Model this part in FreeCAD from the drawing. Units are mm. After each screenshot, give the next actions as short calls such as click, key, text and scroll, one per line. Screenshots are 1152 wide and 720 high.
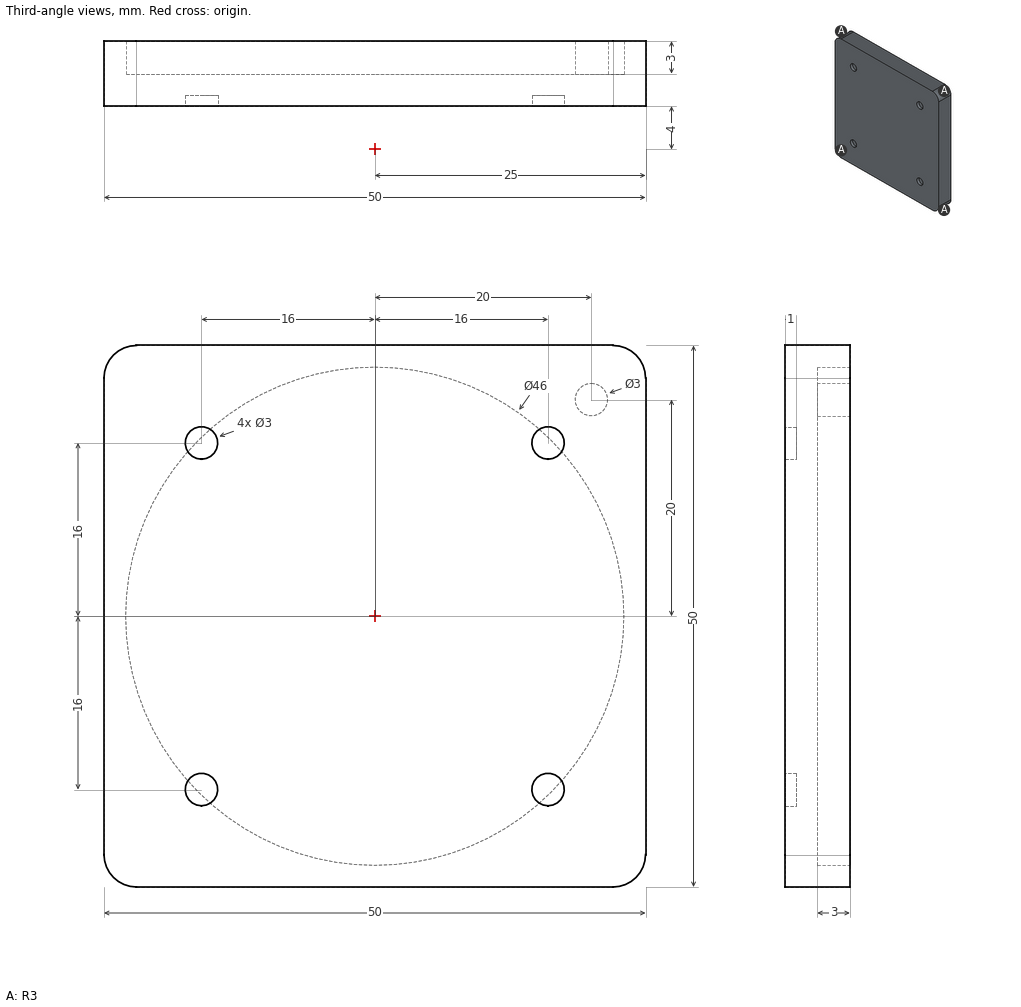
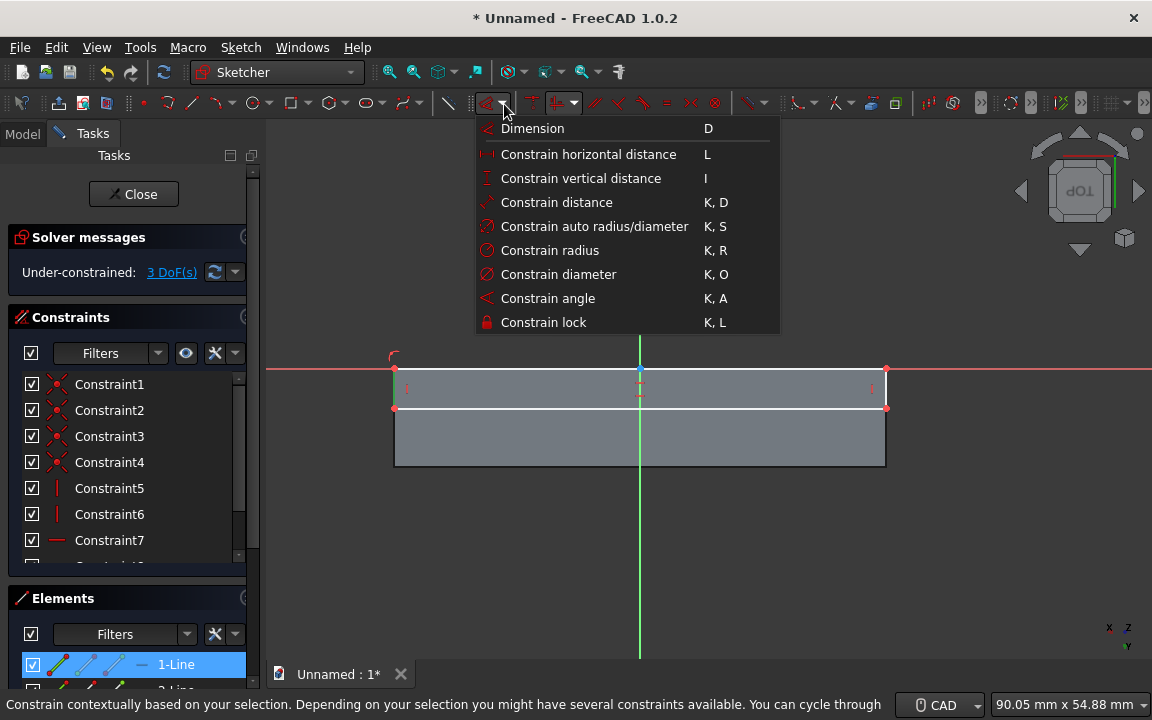
click(628, 178)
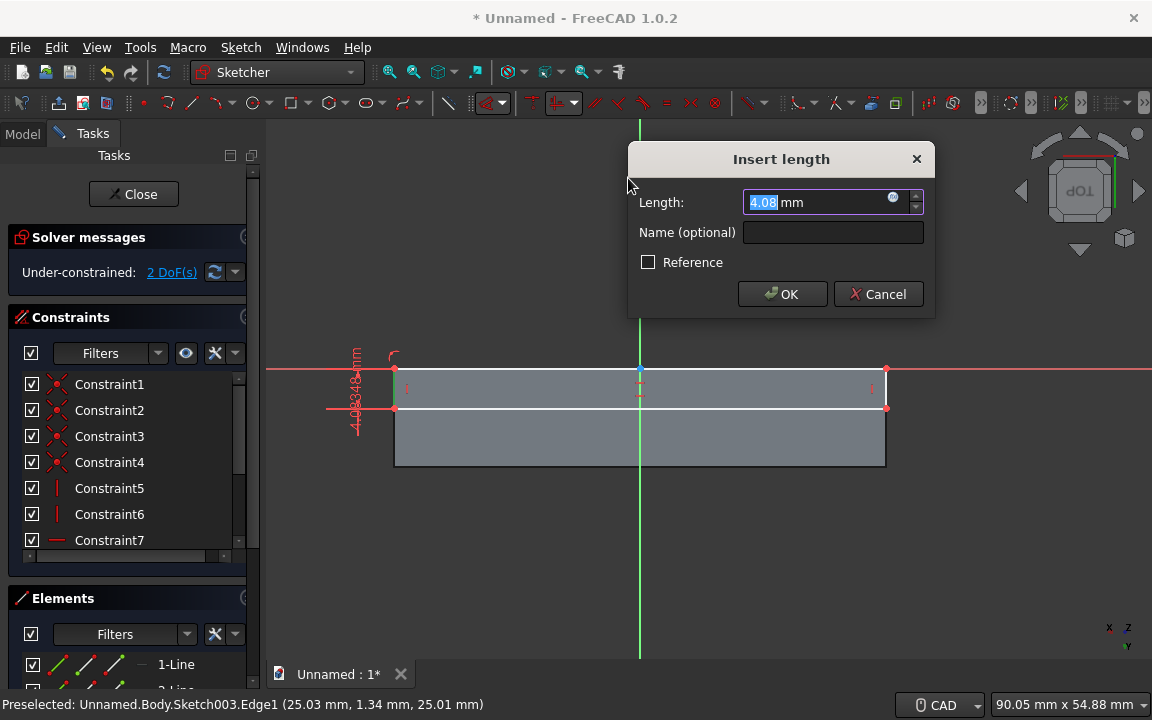
text(4)
key(Return)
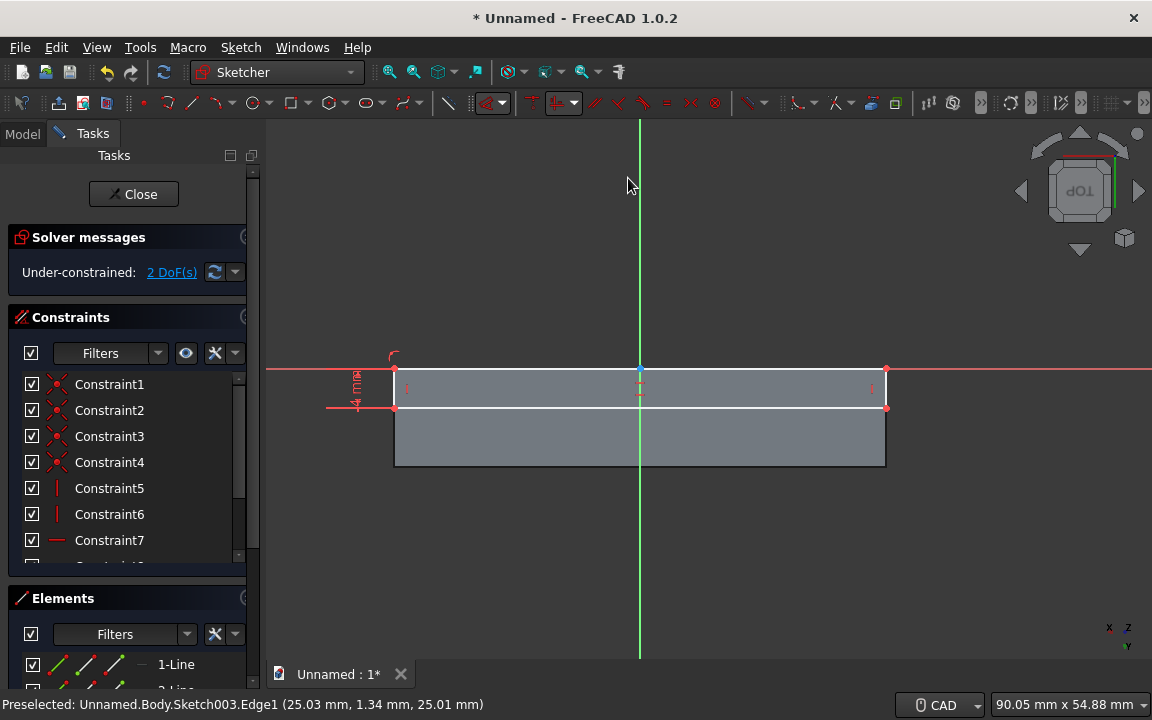
click(542, 408)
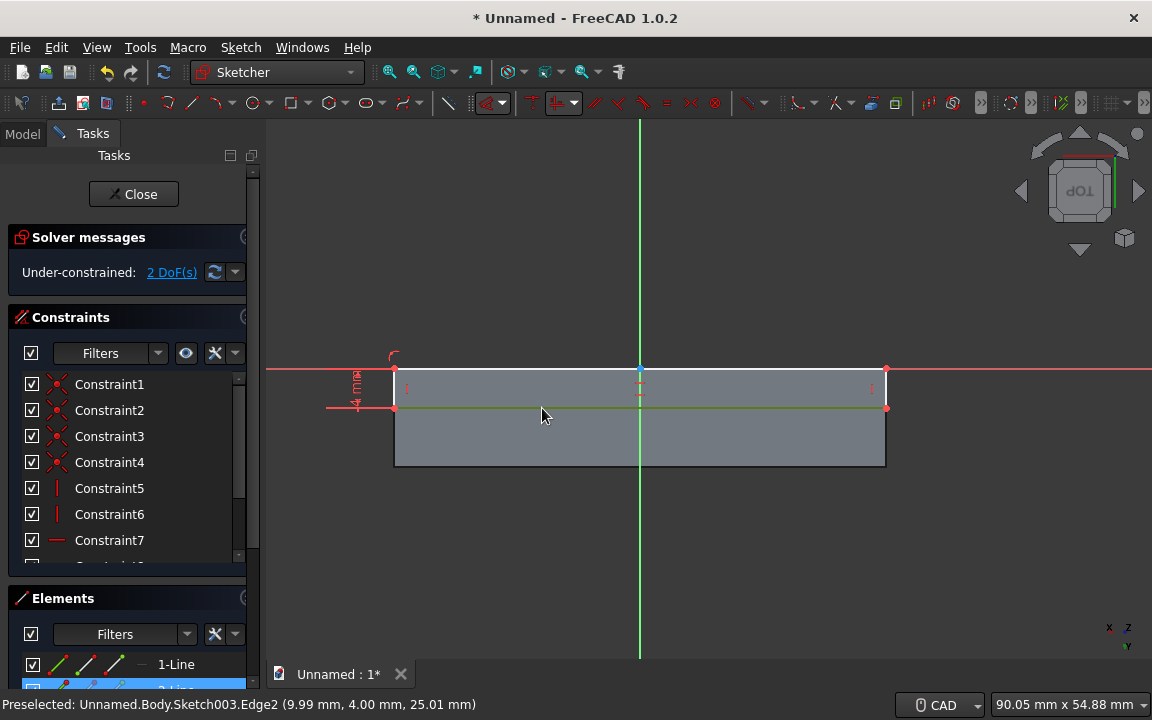
key(l)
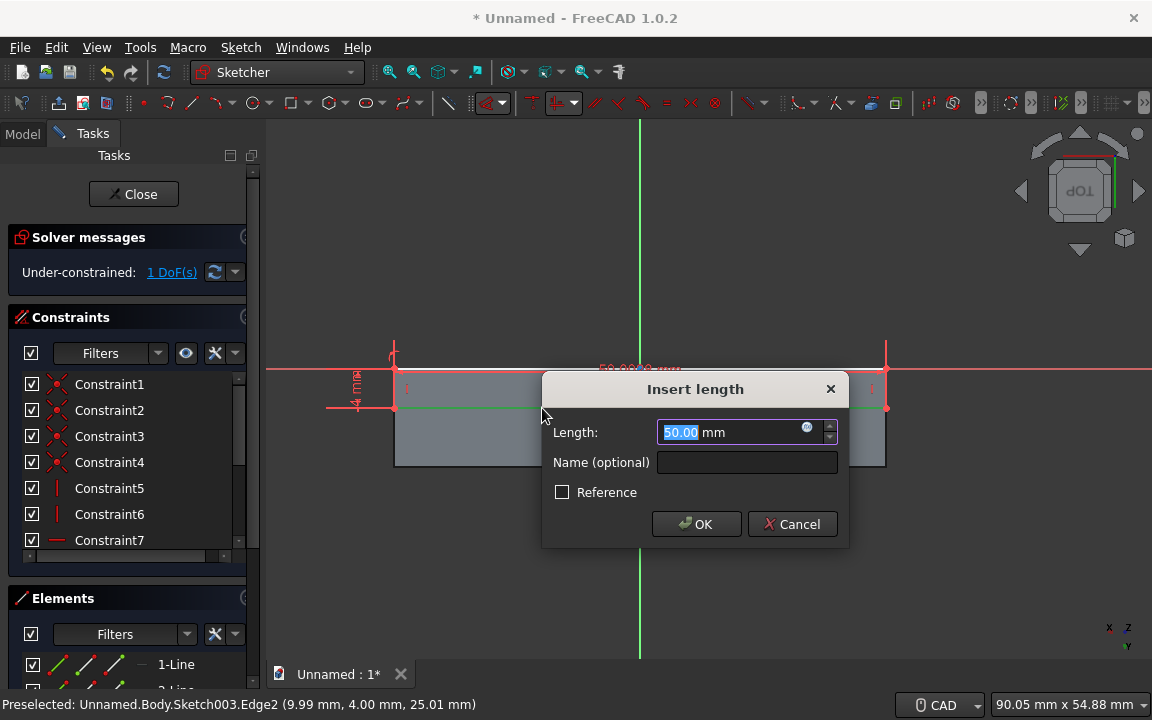
text(50)
key(Return)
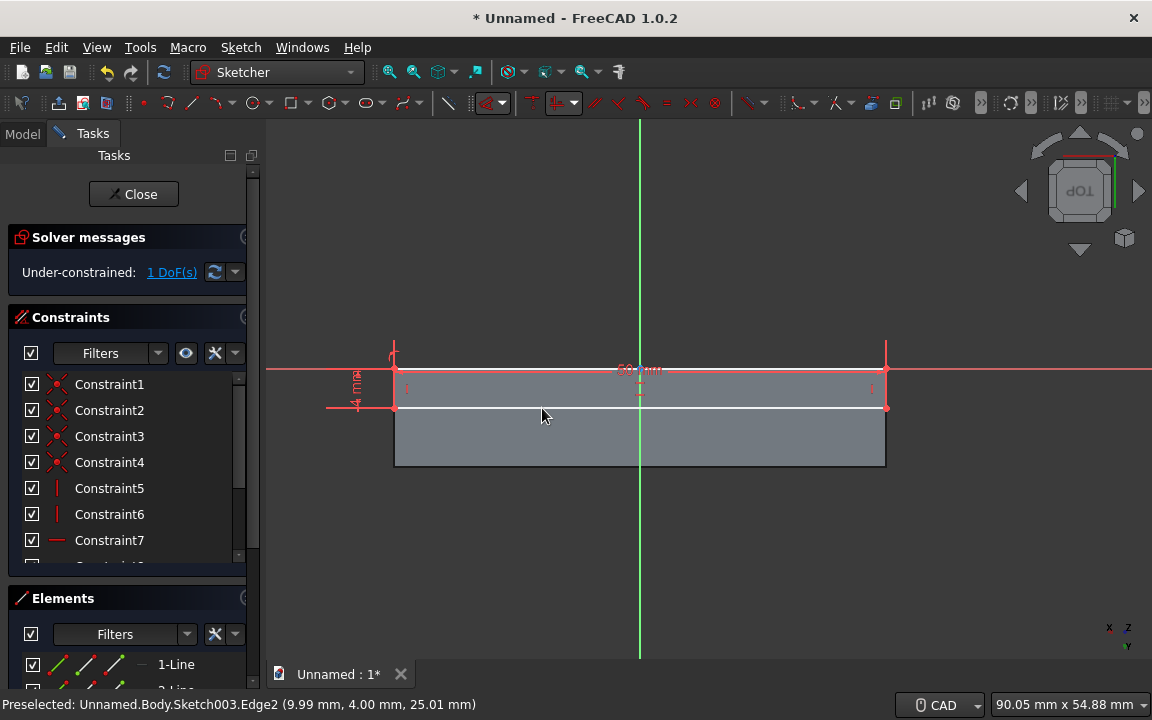
click(394, 369)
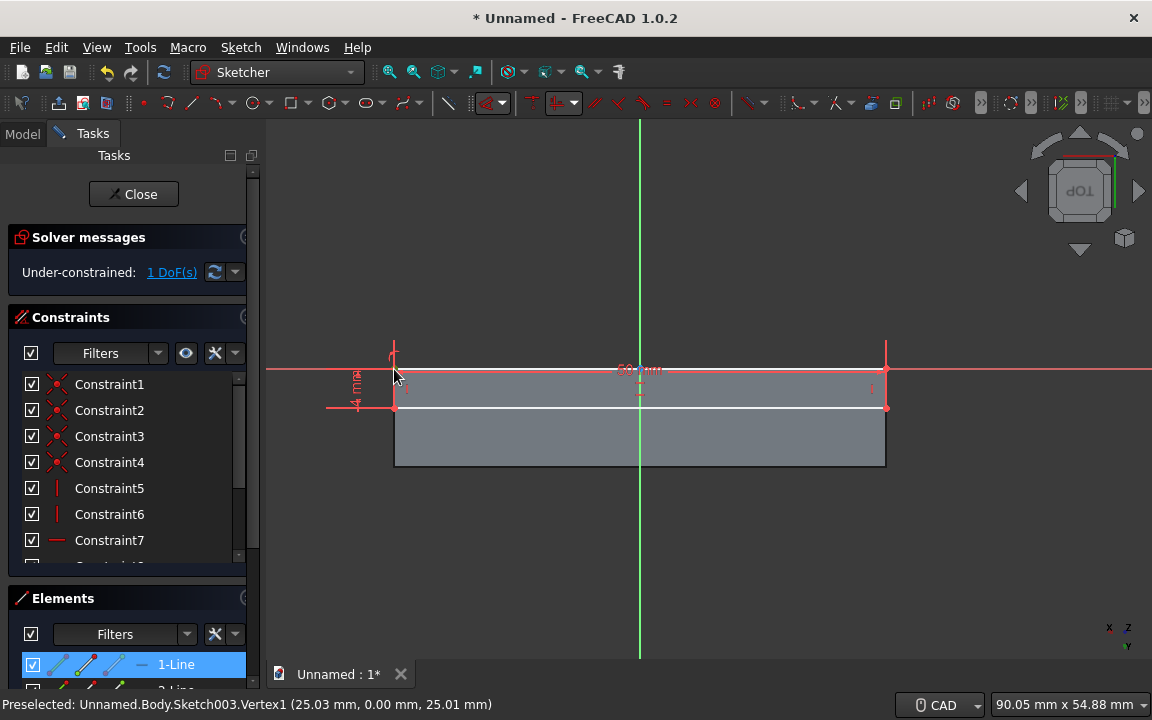
click(504, 104)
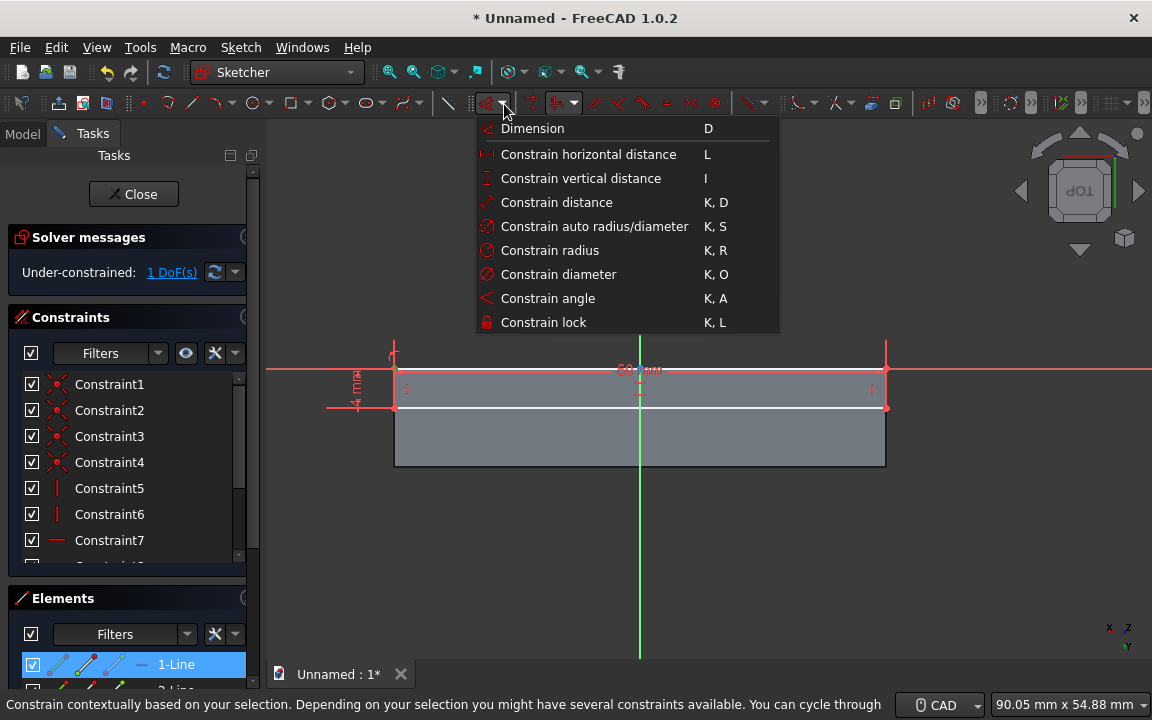
click(628, 154)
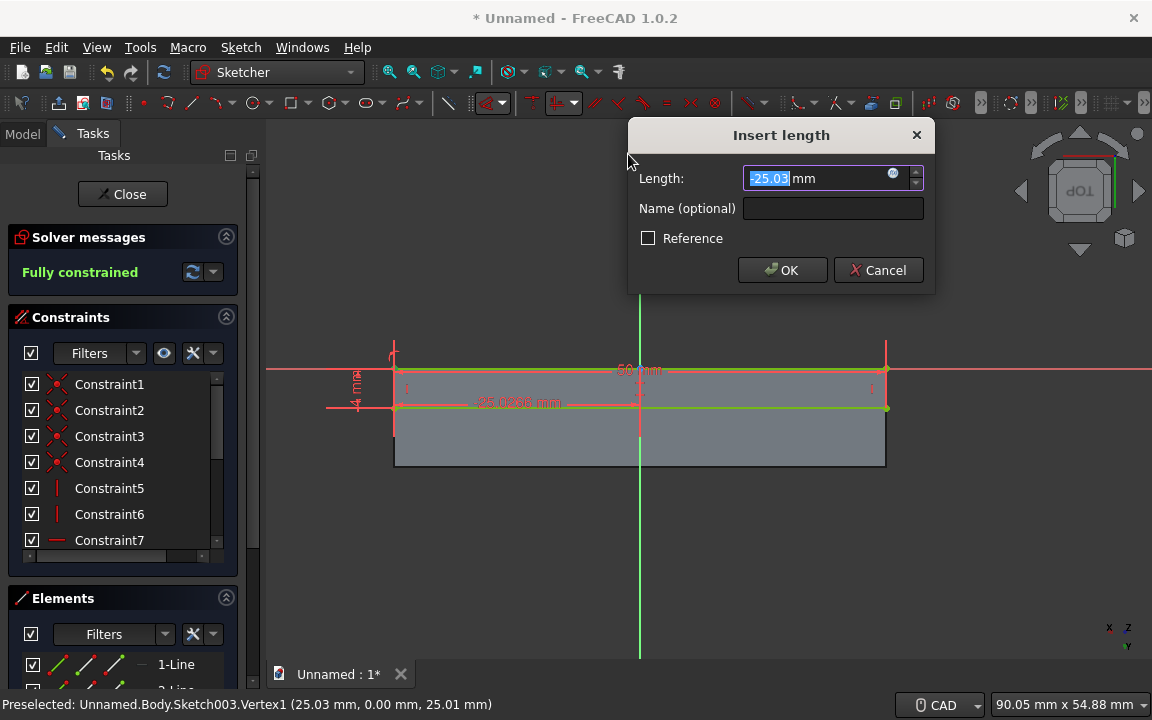
text(-25)
key(Return)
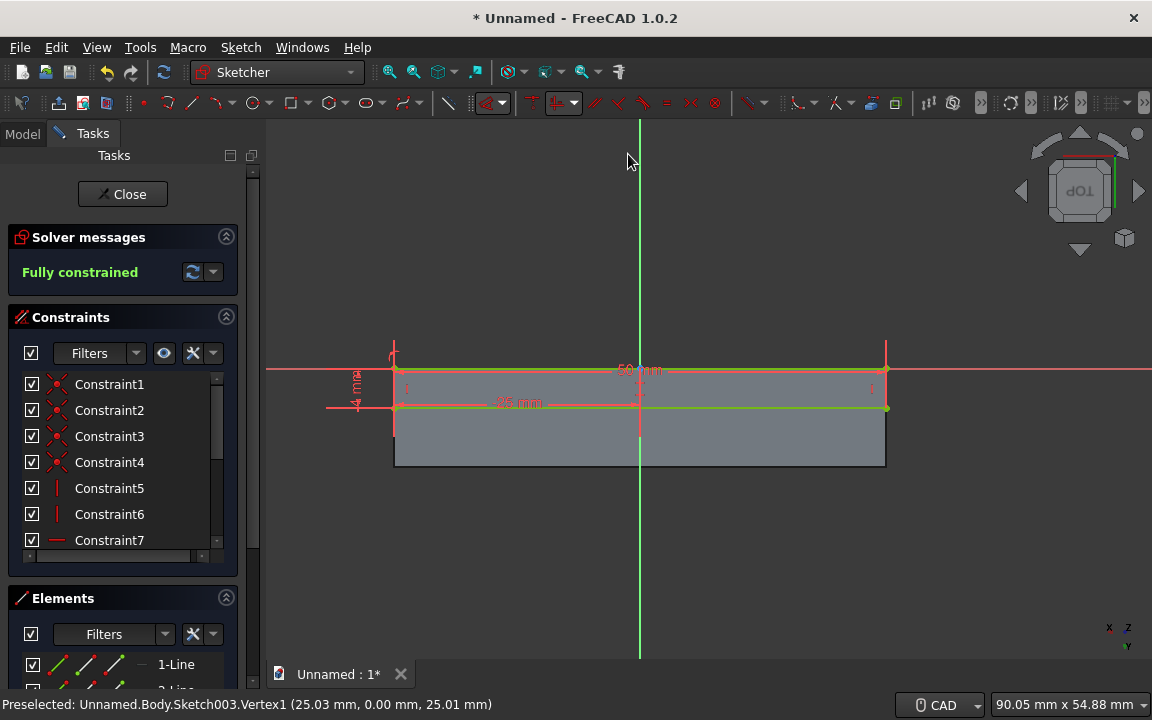
click(123, 194)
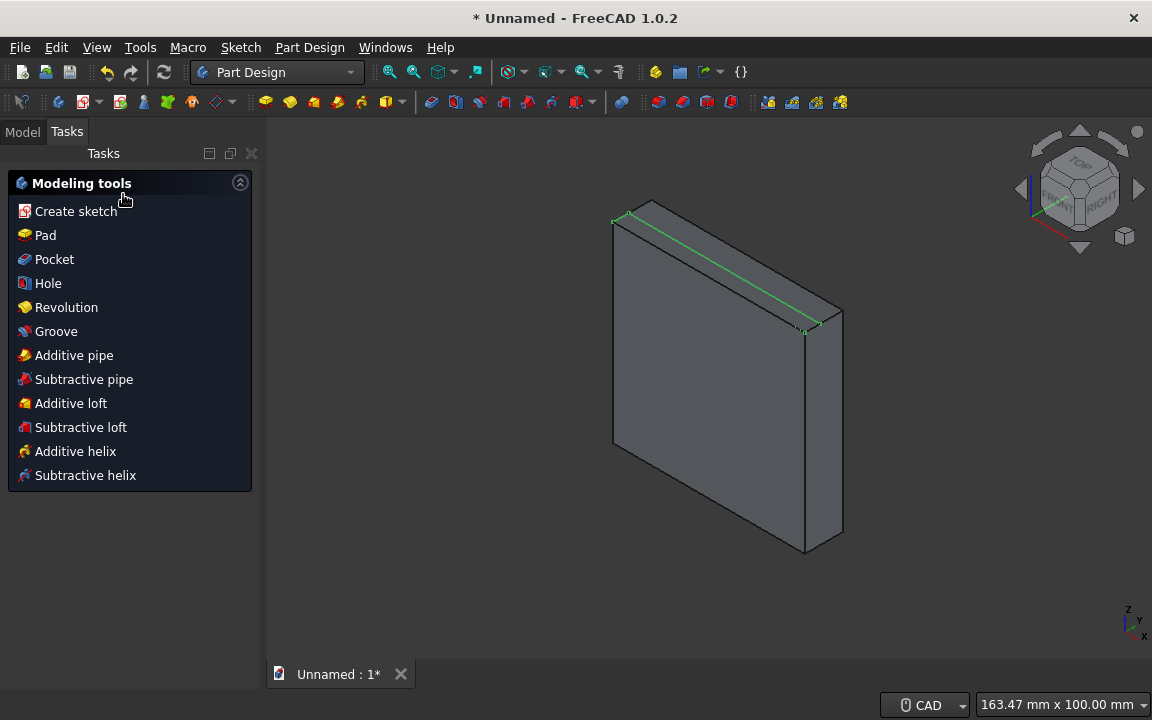
click(432, 102)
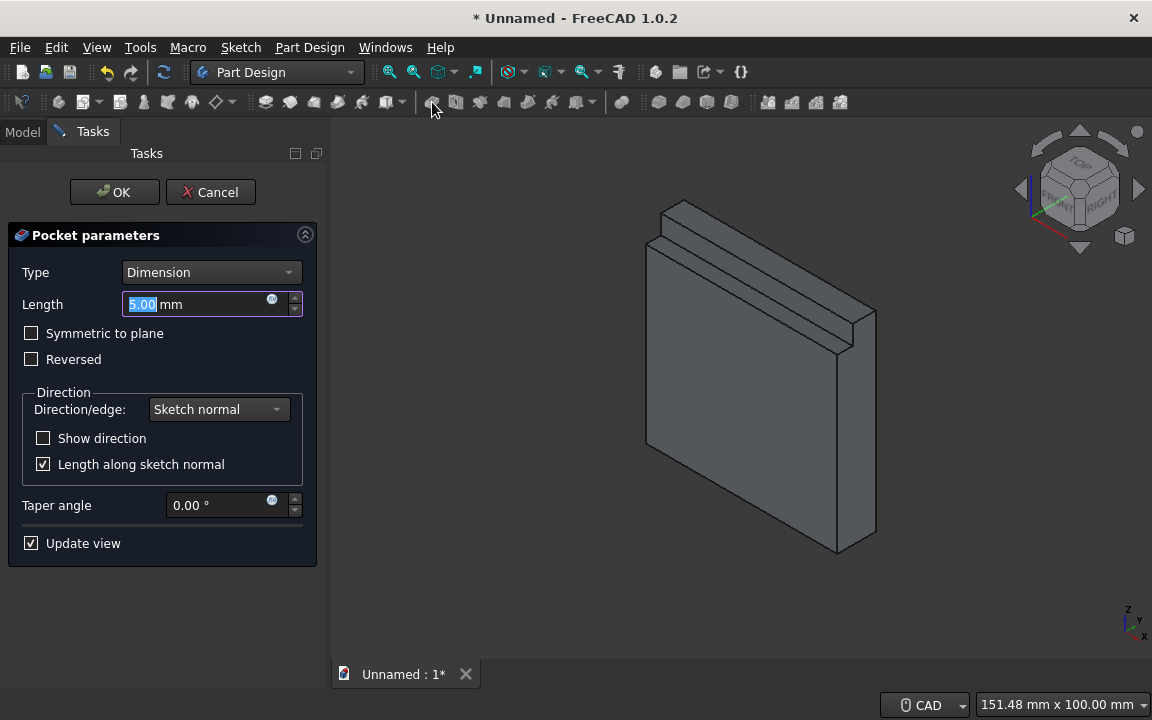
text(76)
key(Tab)